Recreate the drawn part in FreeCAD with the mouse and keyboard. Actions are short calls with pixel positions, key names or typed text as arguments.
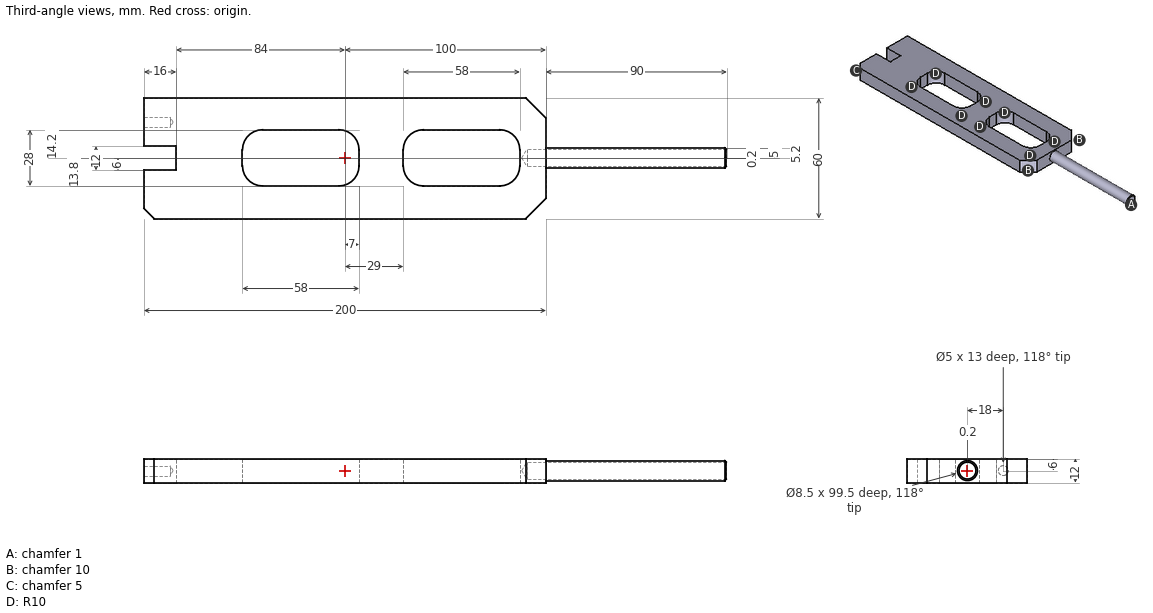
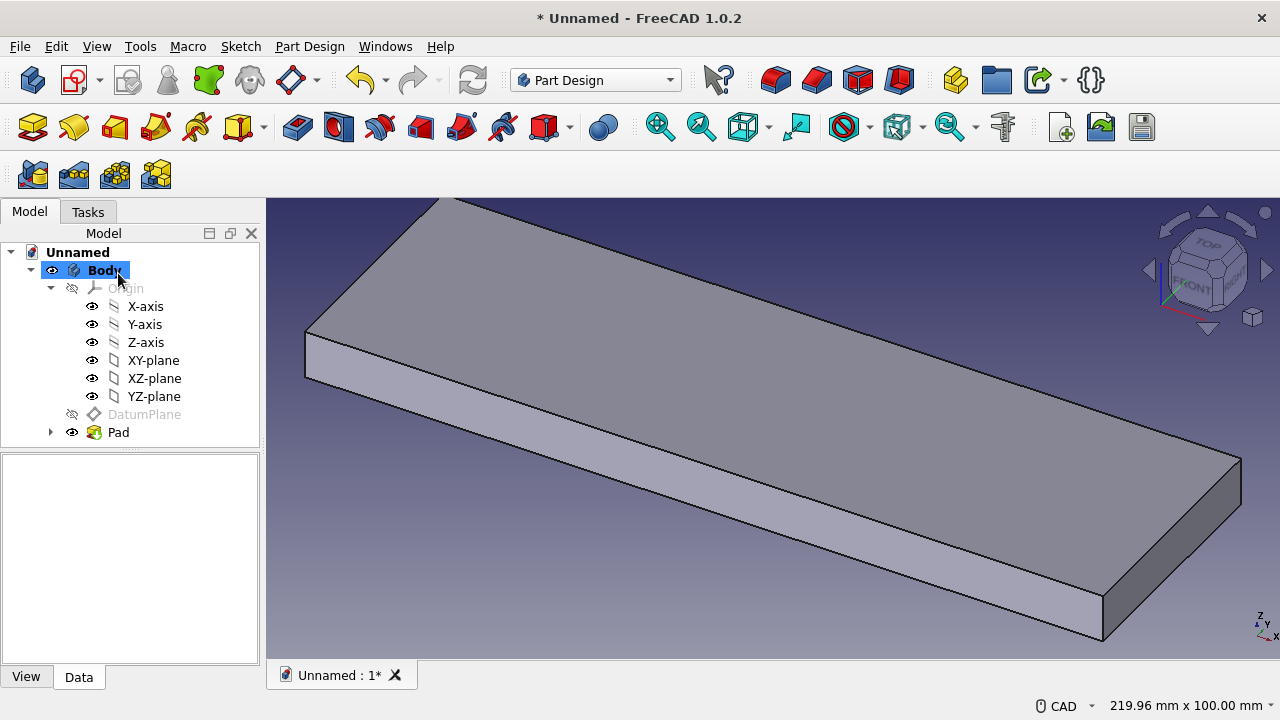
click(661, 128)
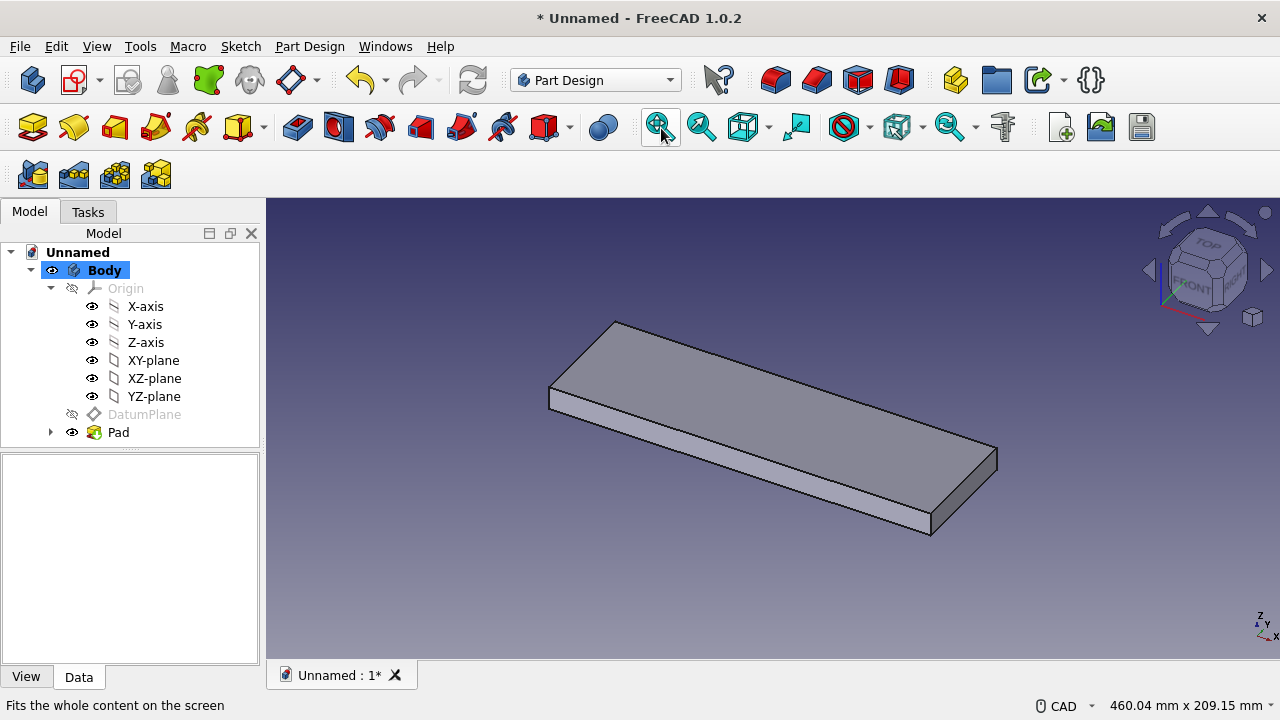
key(5)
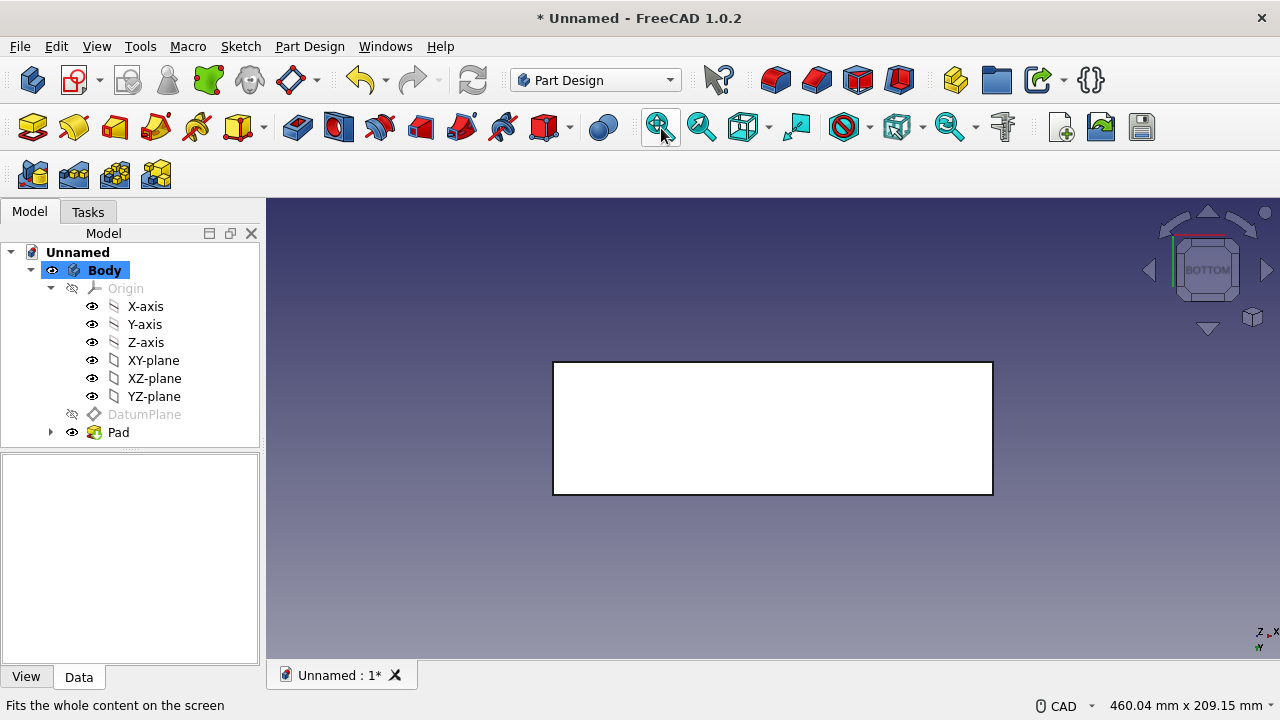
click(661, 128)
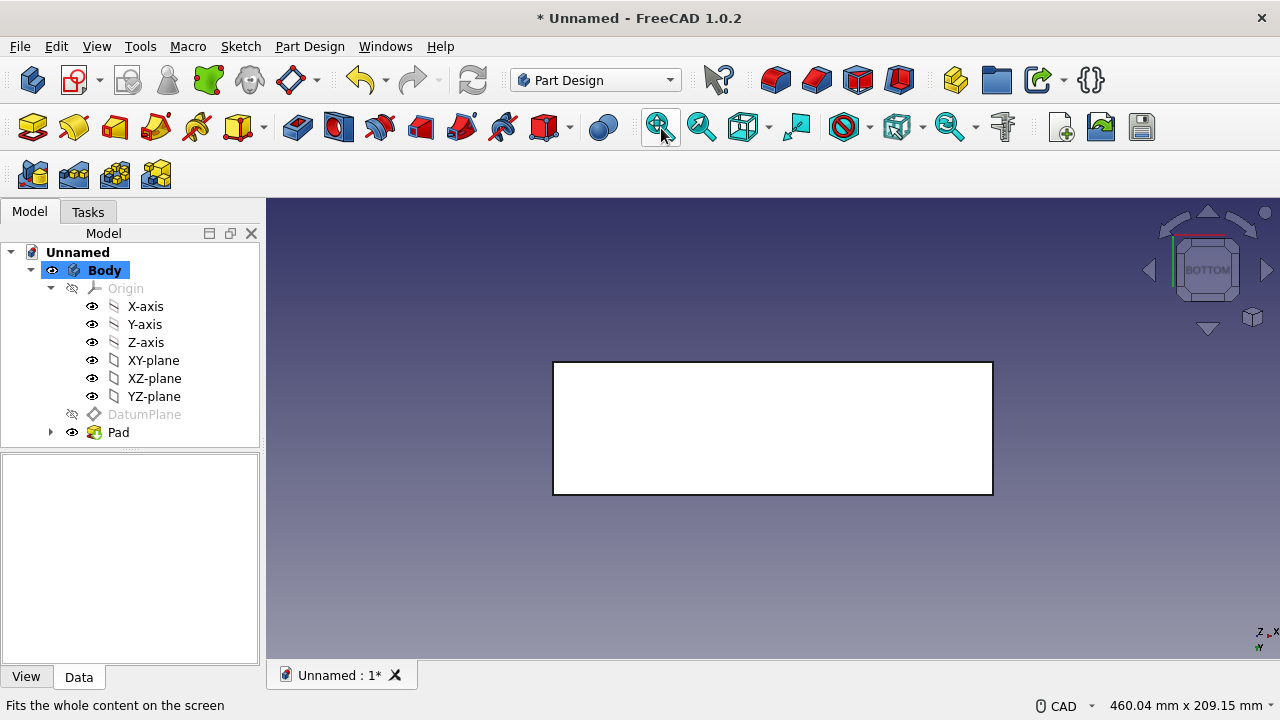
click(899, 427)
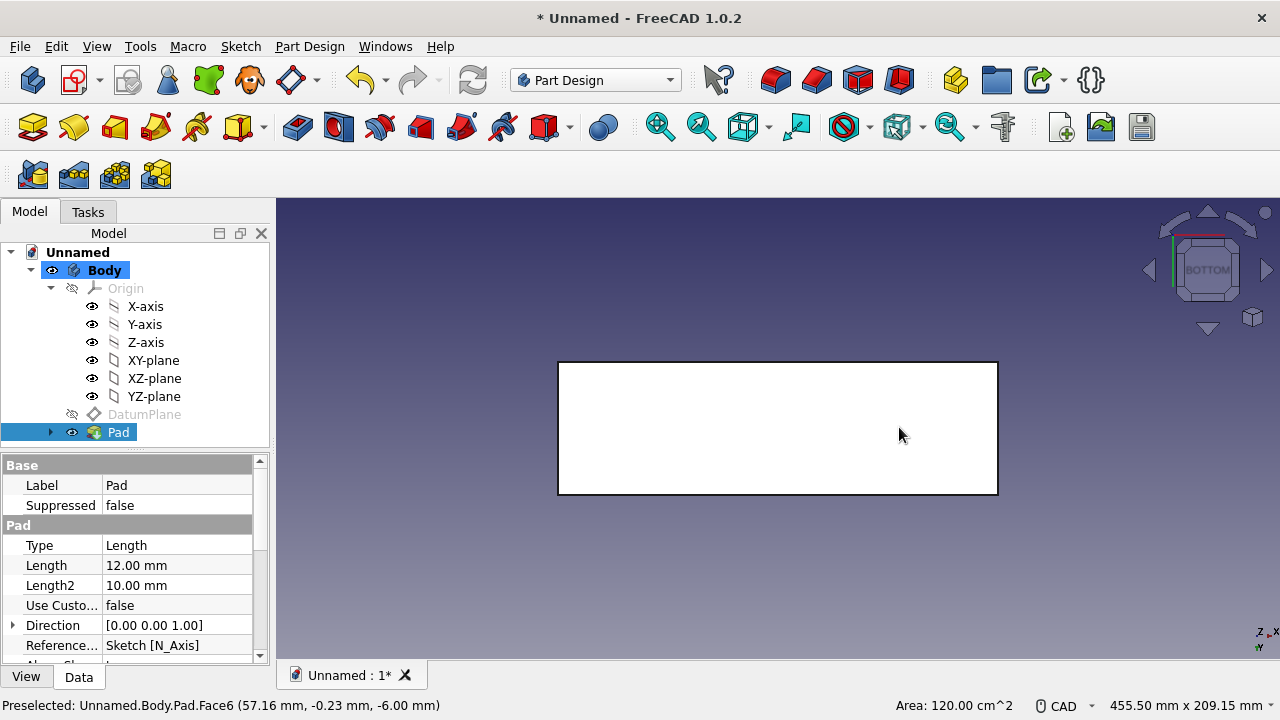
click(74, 80)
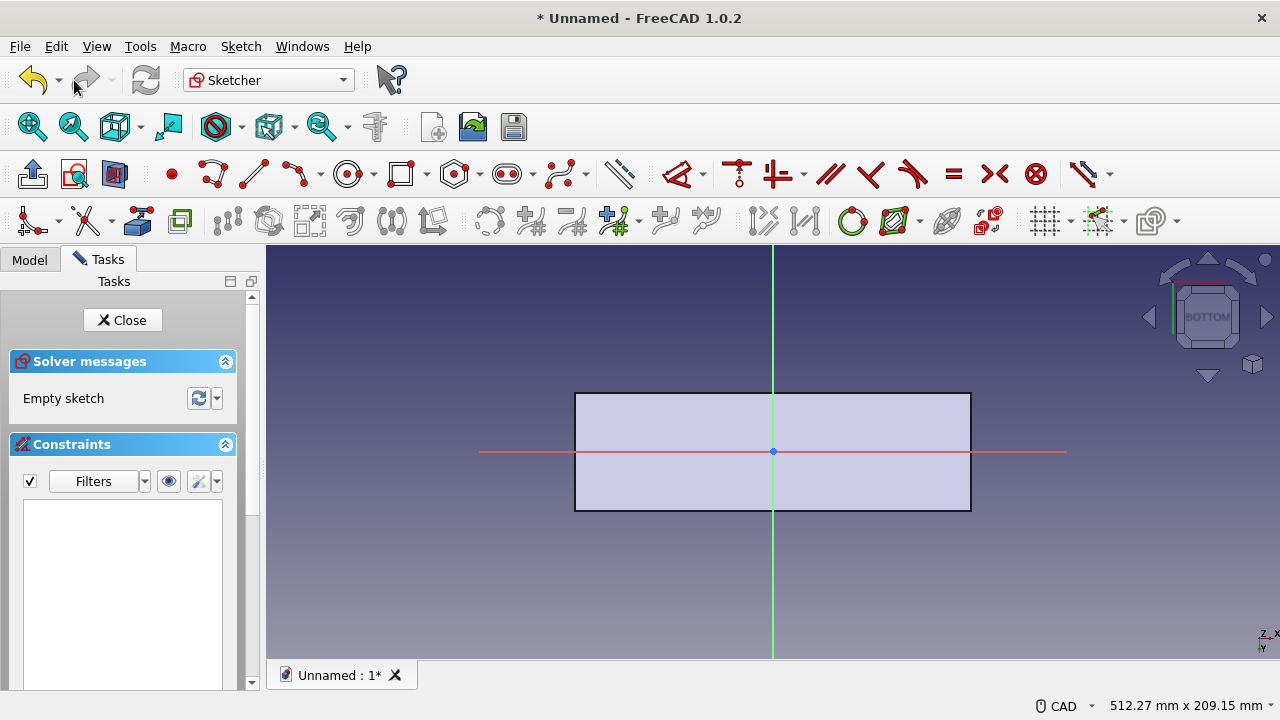
scroll(580, 452, up, 12)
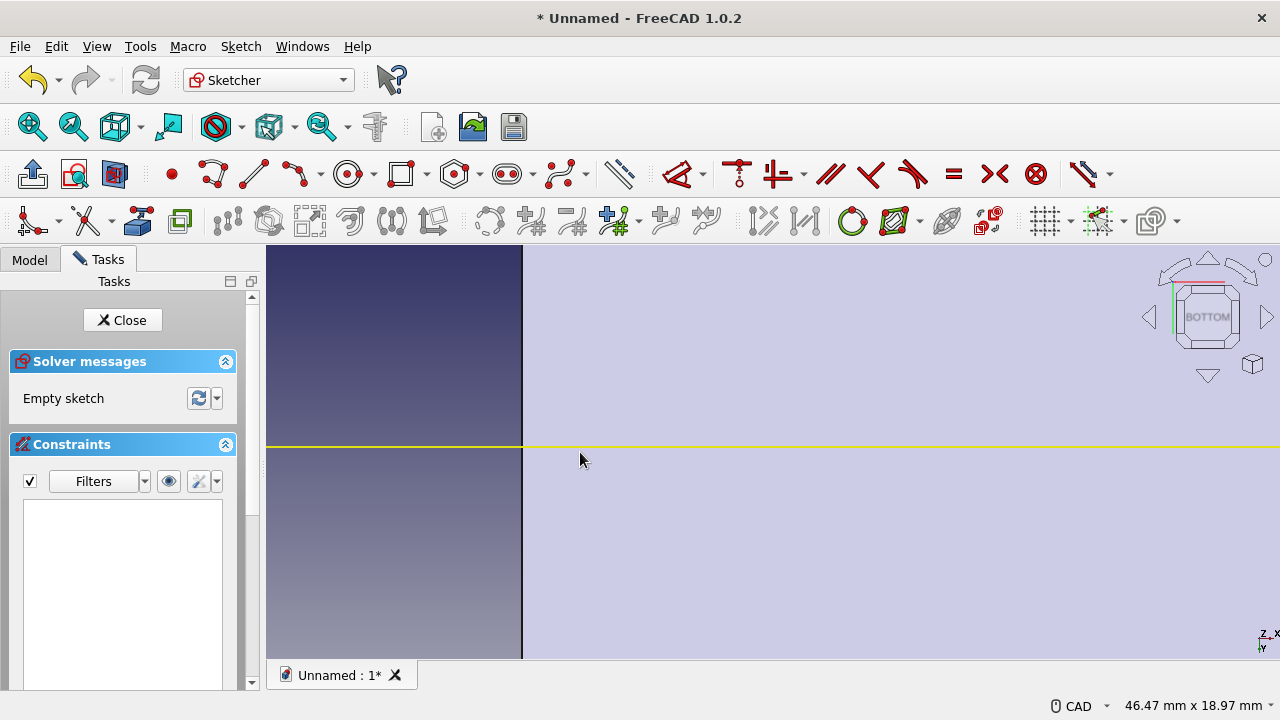
key(g)
key(r)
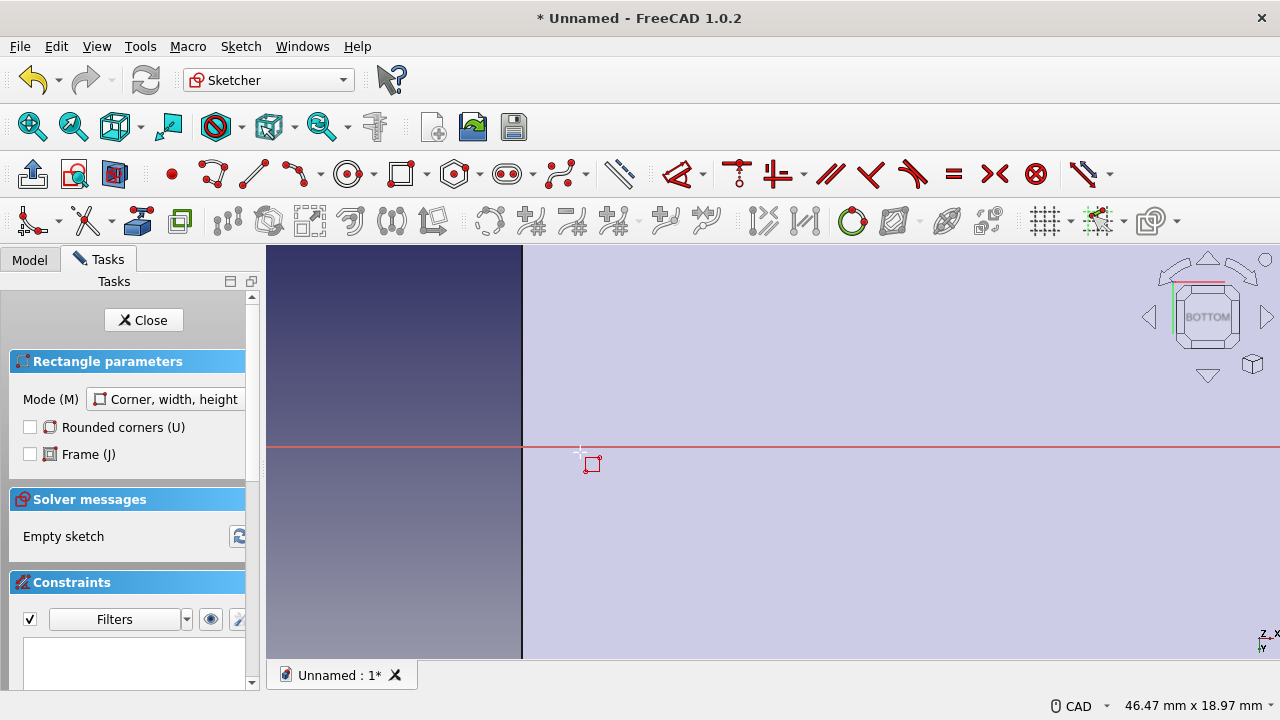
click(522, 316)
move(872, 578)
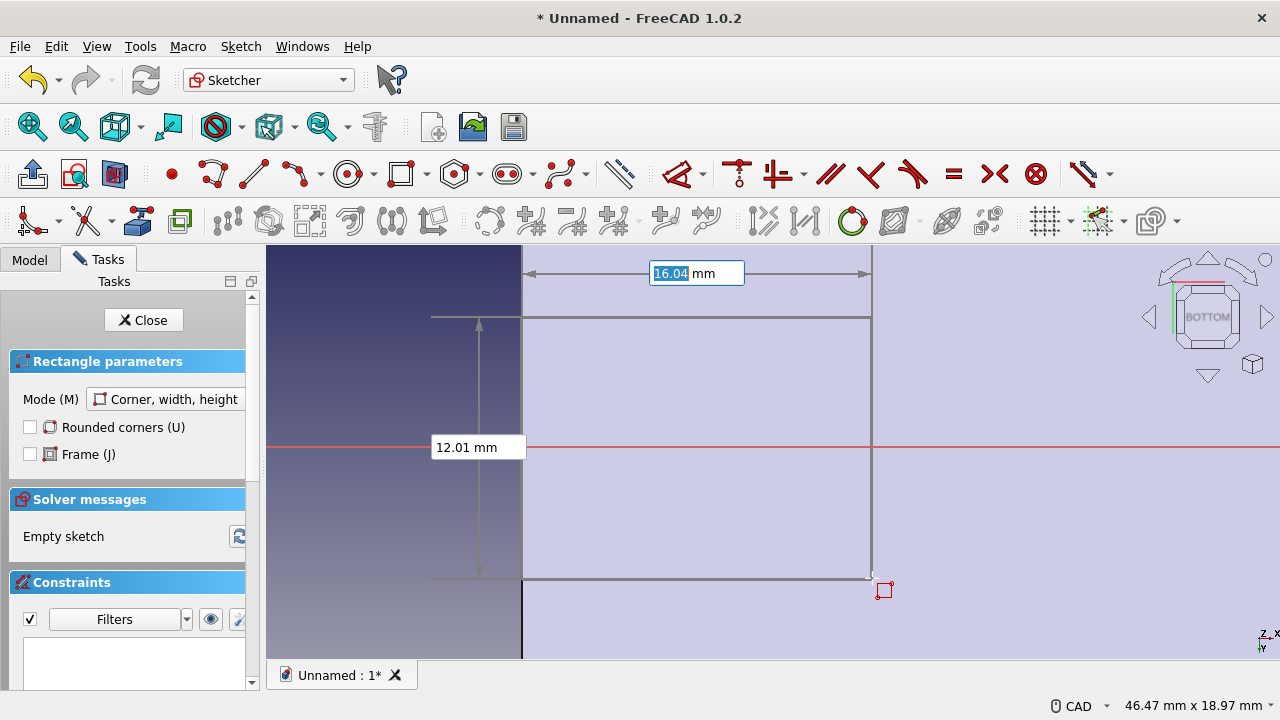
text(16)
key(Tab)
text(12)
key(Return)
key(Escape)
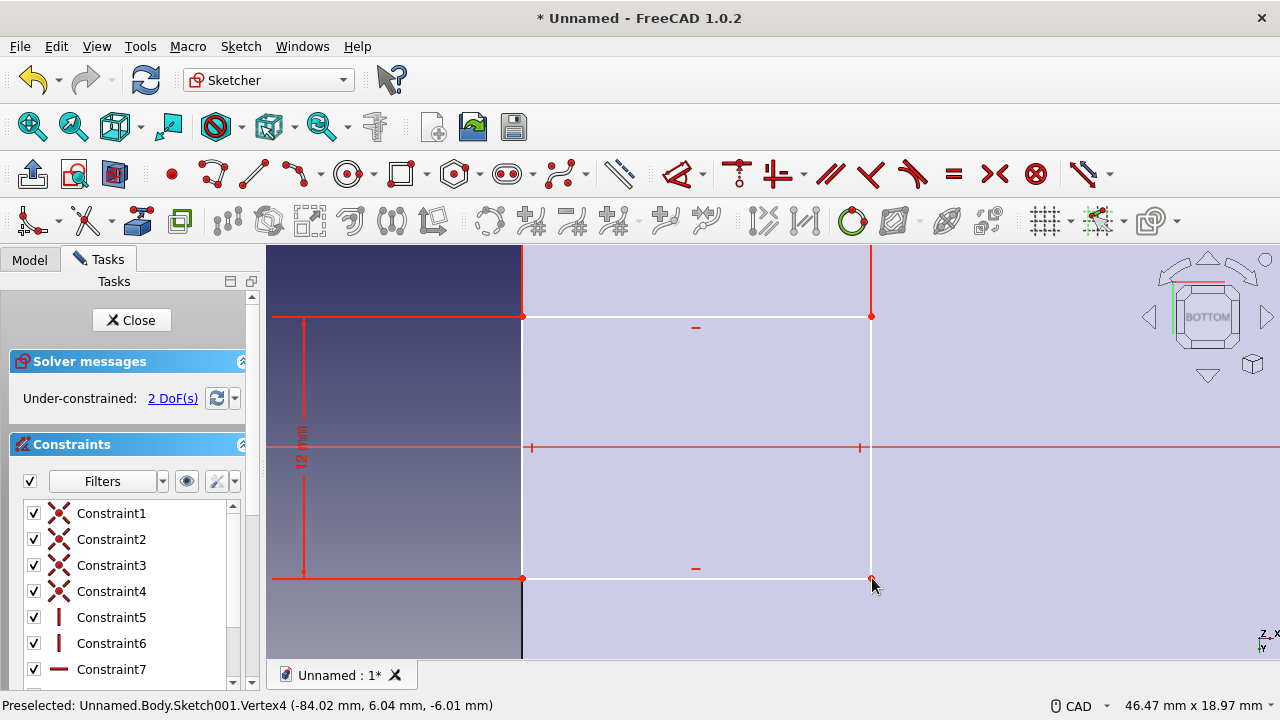
click(522, 317)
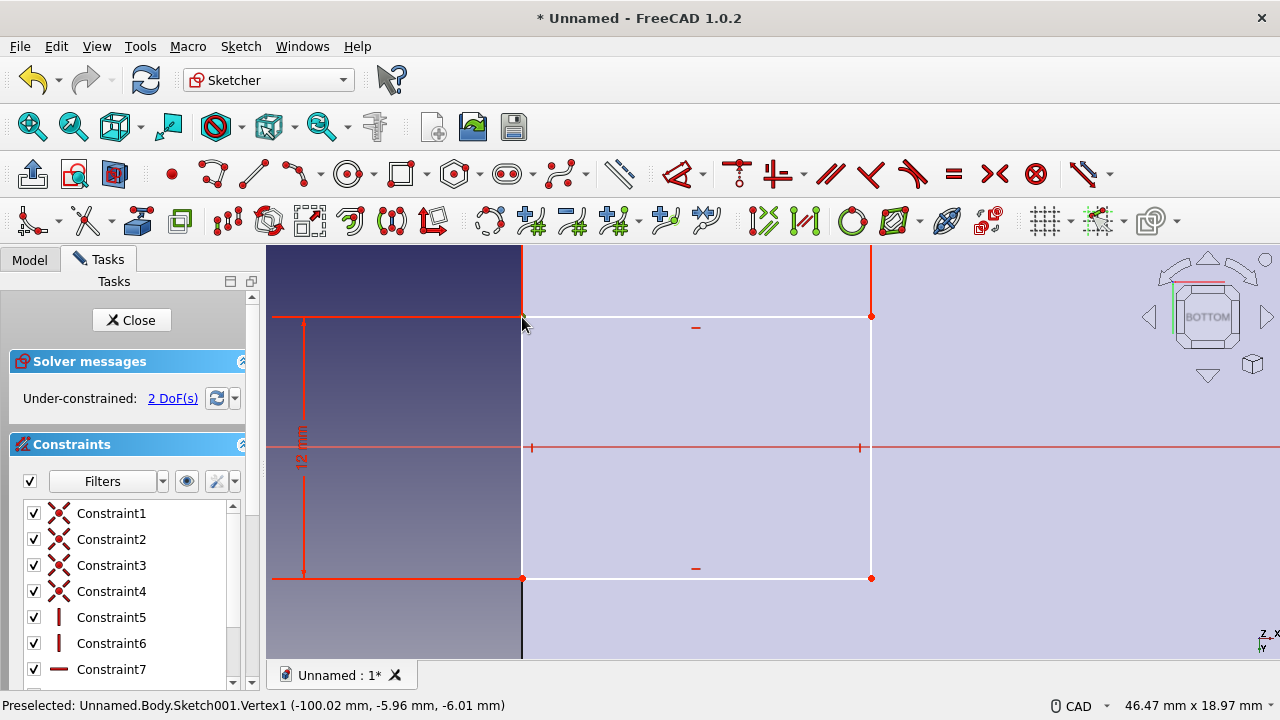
click(702, 174)